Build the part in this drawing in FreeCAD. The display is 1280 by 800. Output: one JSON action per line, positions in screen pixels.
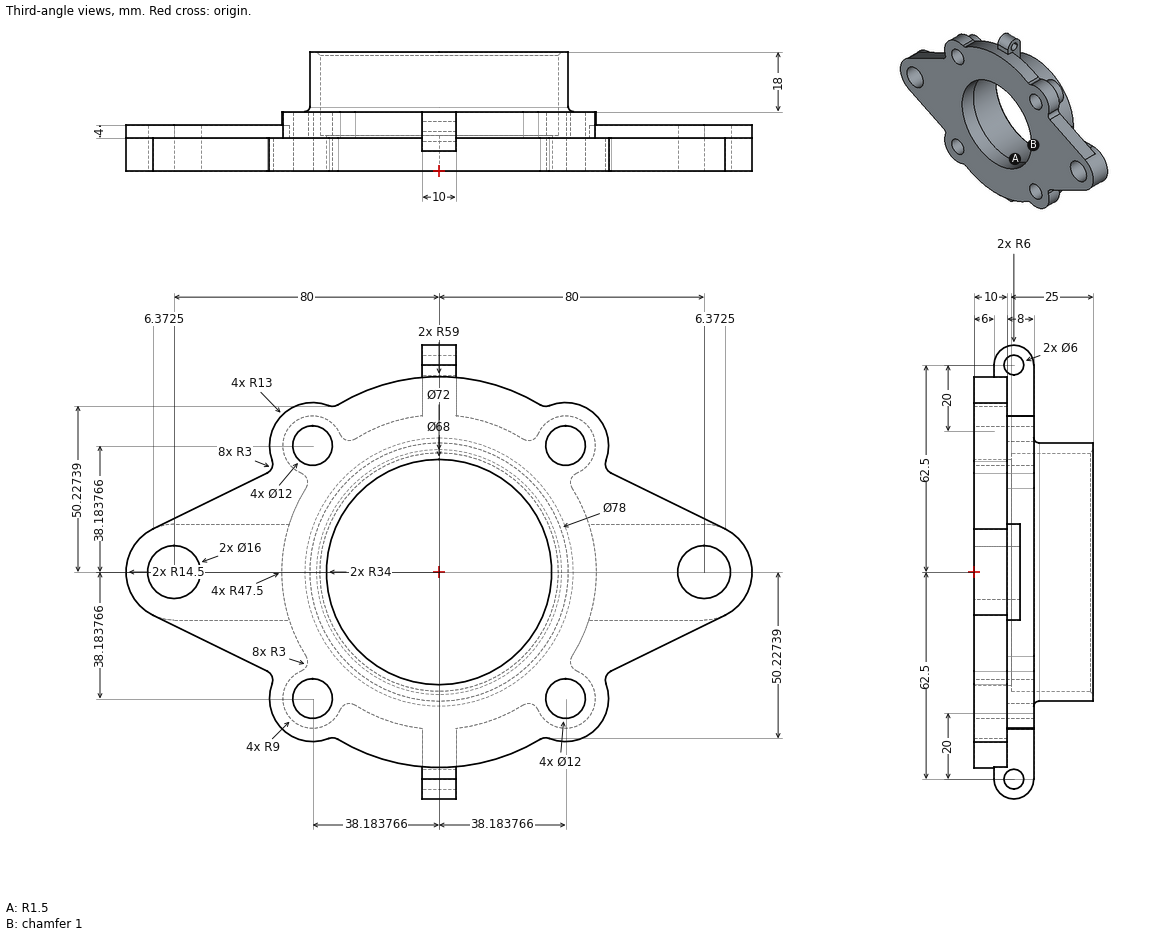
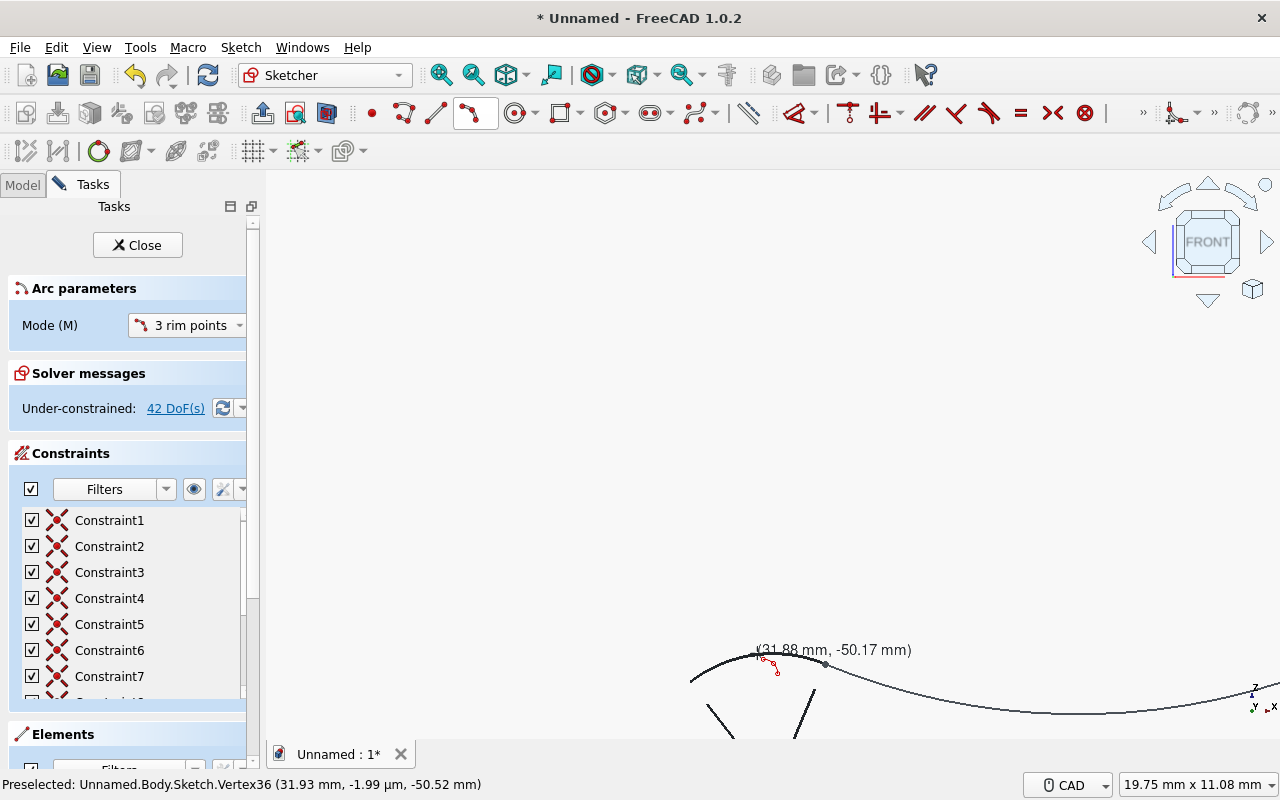
{"action": "left_click", "coordinate": [755, 648]}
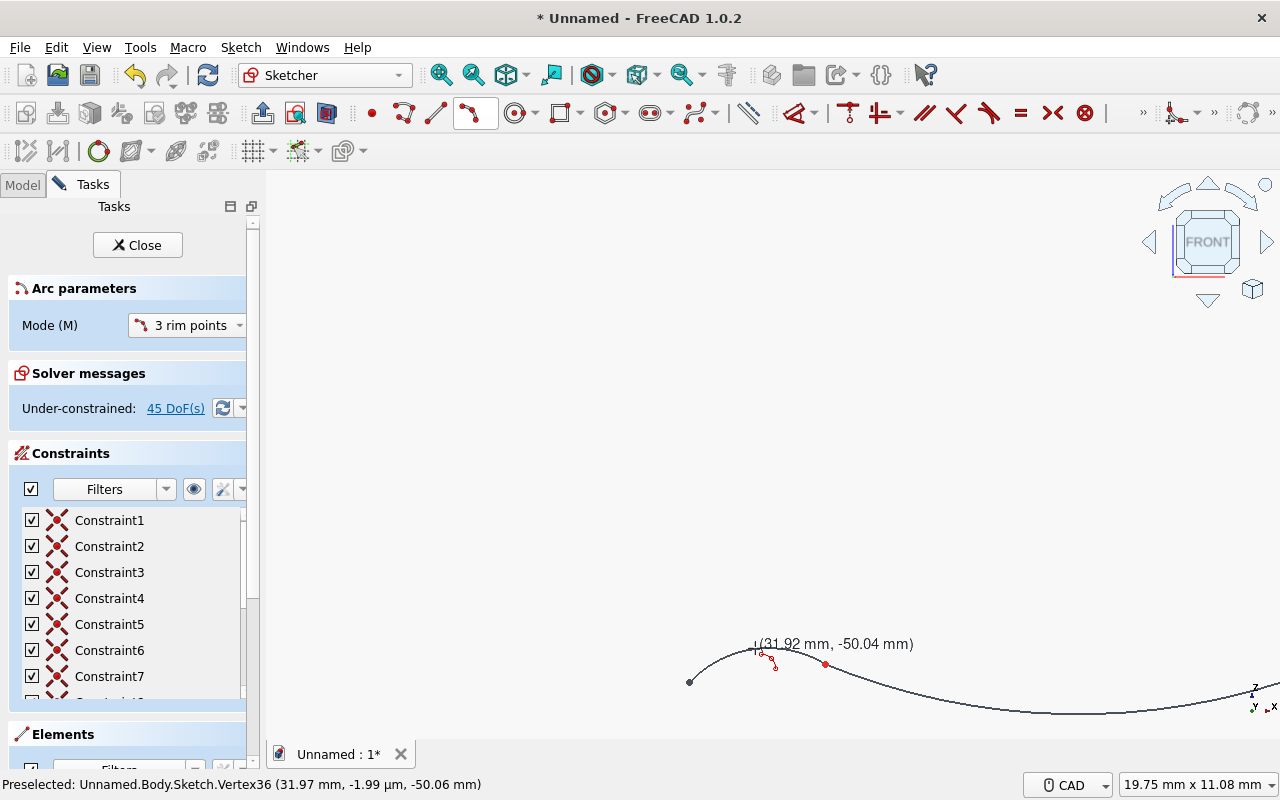
{"action": "scroll", "coordinate": [807, 608], "scroll_direction": "down", "scroll_amount": 14}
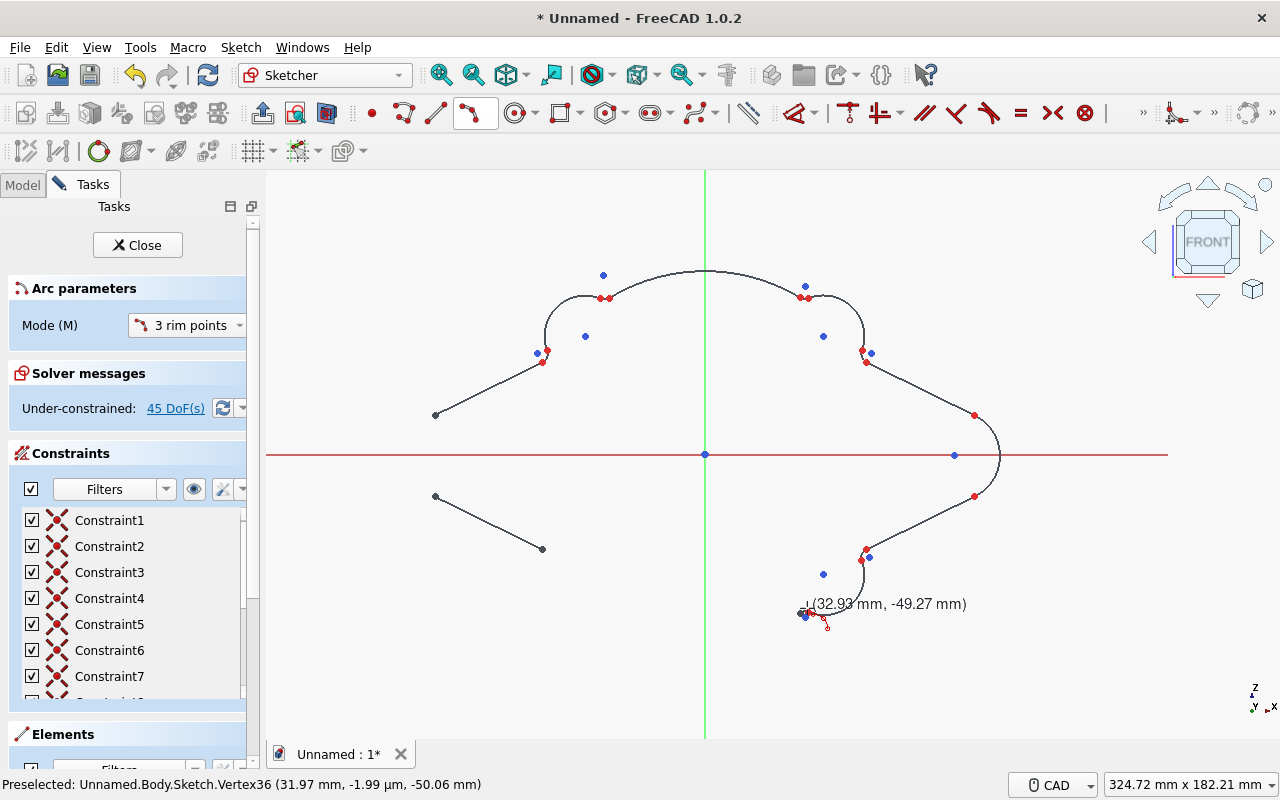
{"action": "scroll", "coordinate": [800, 612], "scroll_direction": "up", "scroll_amount": 4}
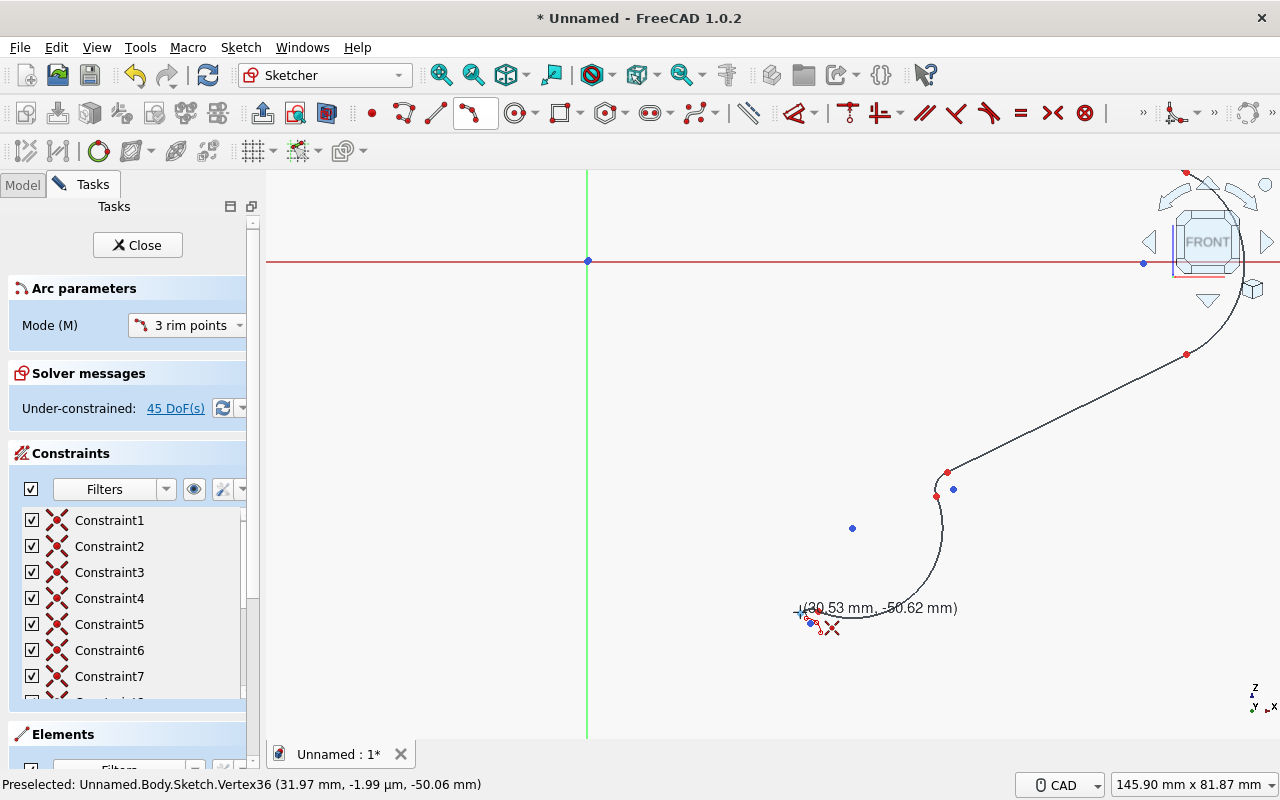
{"action": "left_click", "coordinate": [800, 614]}
{"action": "left_click", "coordinate": [374, 612]}
{"action": "left_click", "coordinate": [543, 669]}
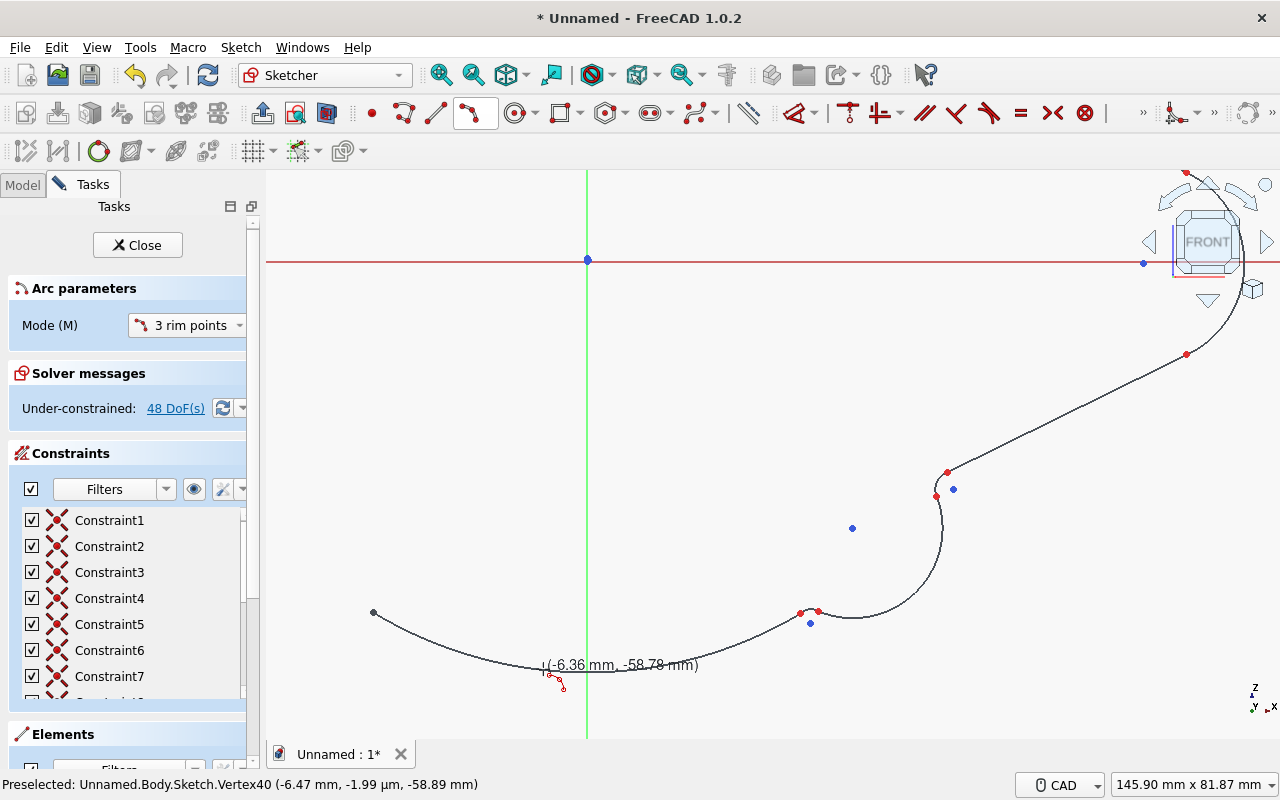
{"action": "left_click", "coordinate": [374, 613]}
{"action": "left_click", "coordinate": [356, 611]}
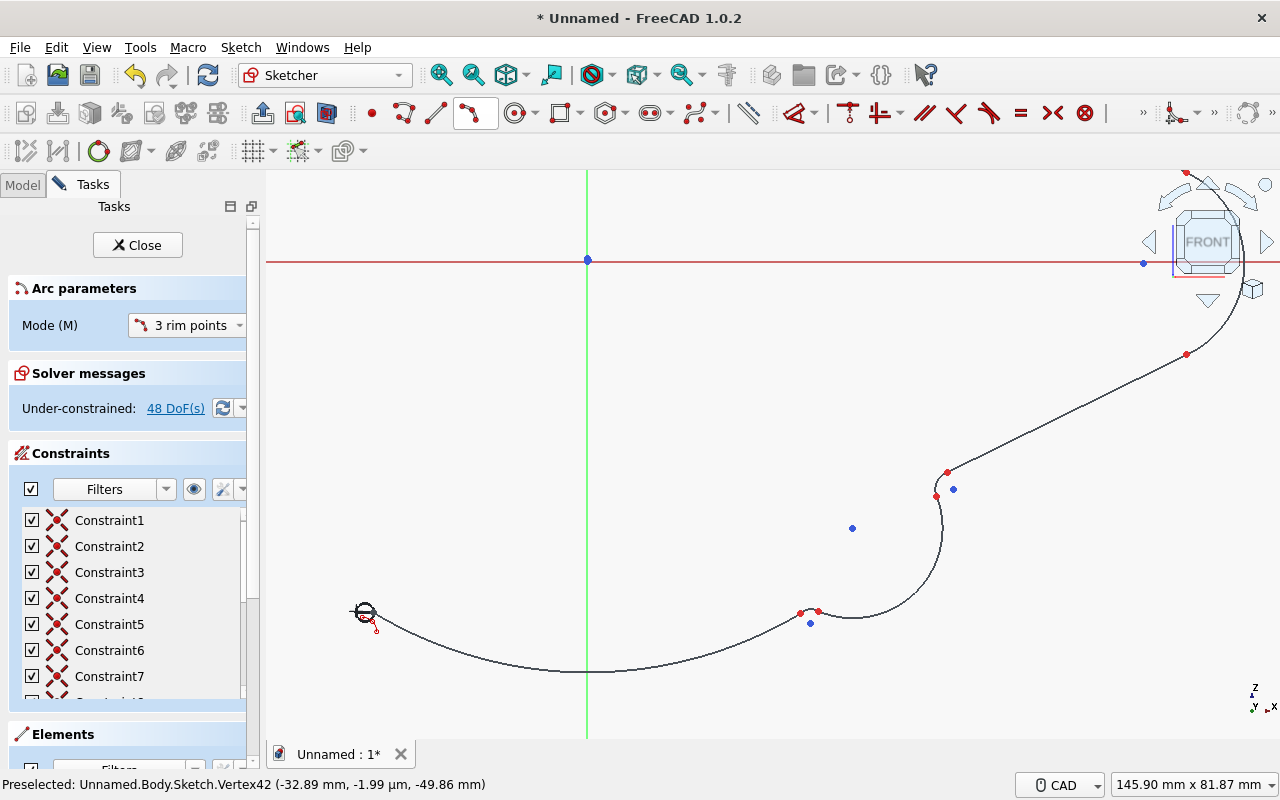
{"action": "scroll", "coordinate": [365, 609], "scroll_direction": "up", "scroll_amount": 10}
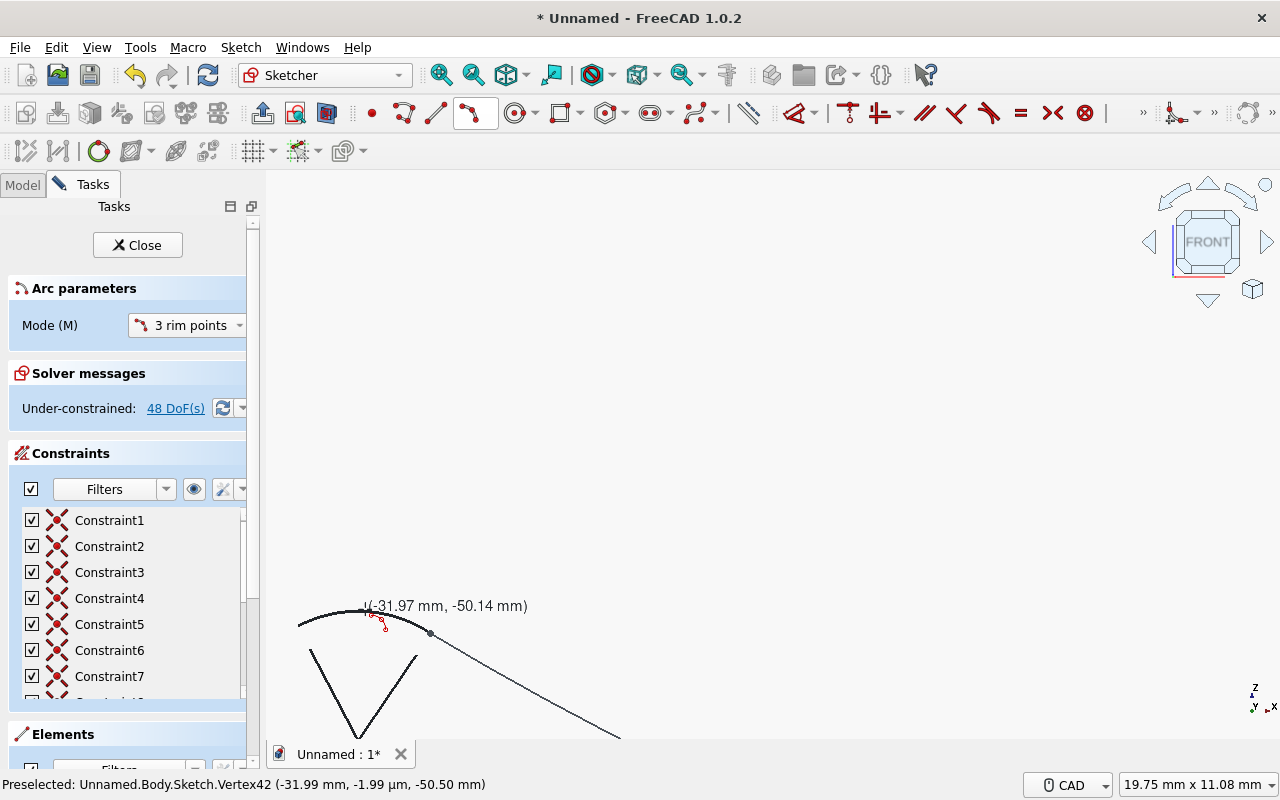
{"action": "left_click", "coordinate": [367, 605]}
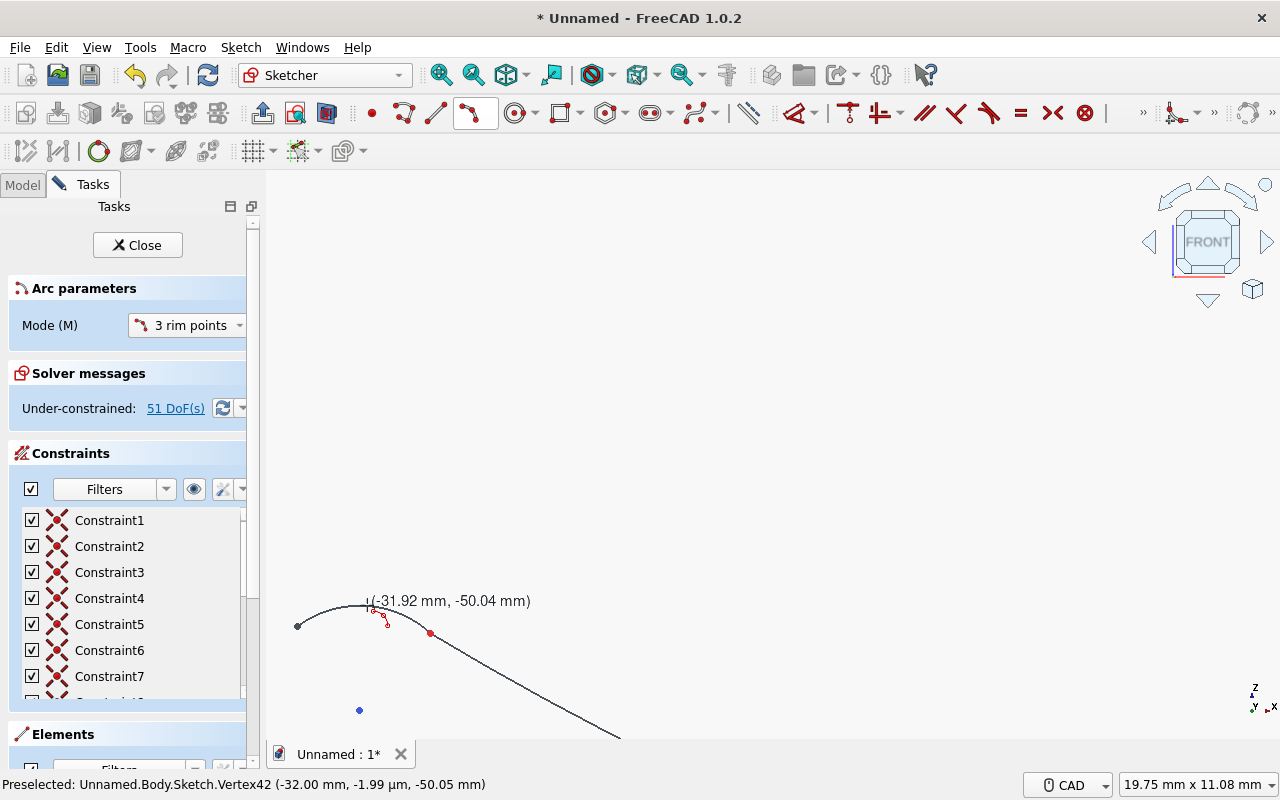
{"action": "scroll", "coordinate": [620, 611], "scroll_direction": "down", "scroll_amount": 14}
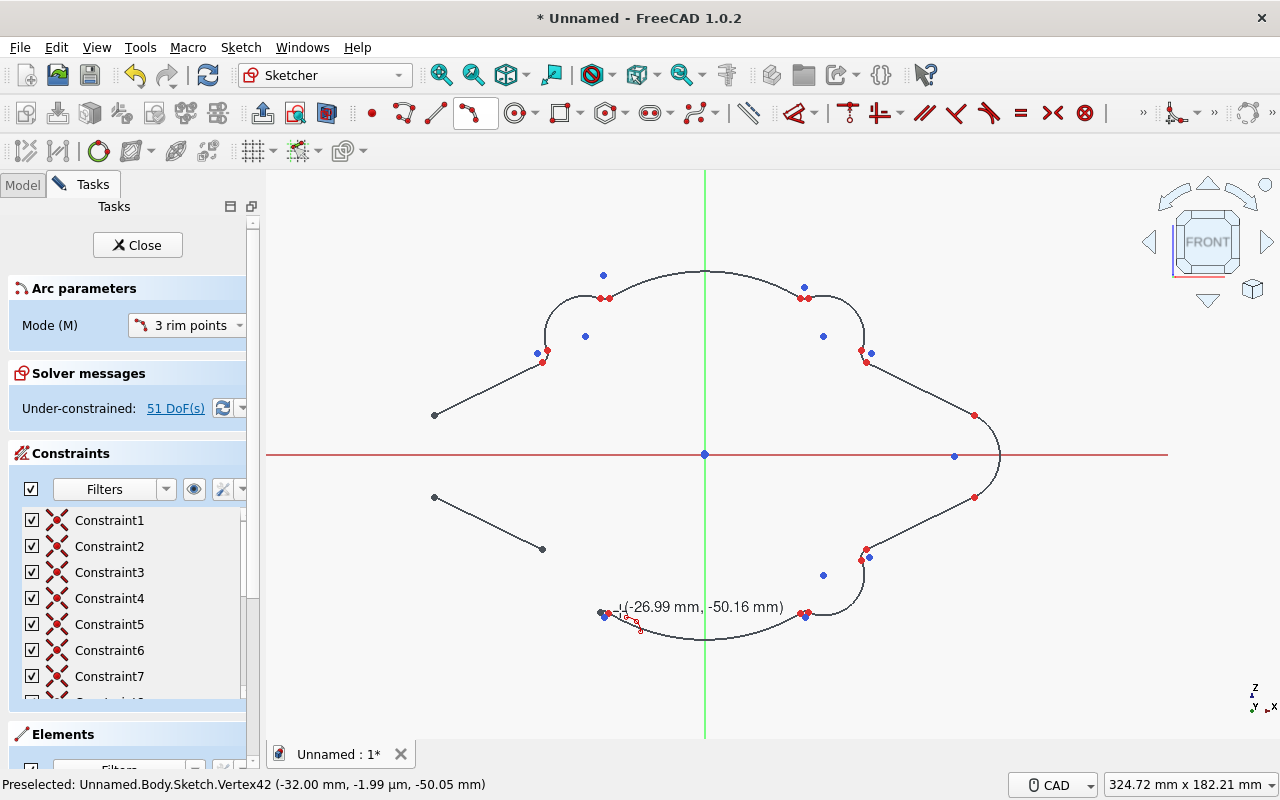
{"action": "scroll", "coordinate": [601, 612], "scroll_direction": "up", "scroll_amount": 4}